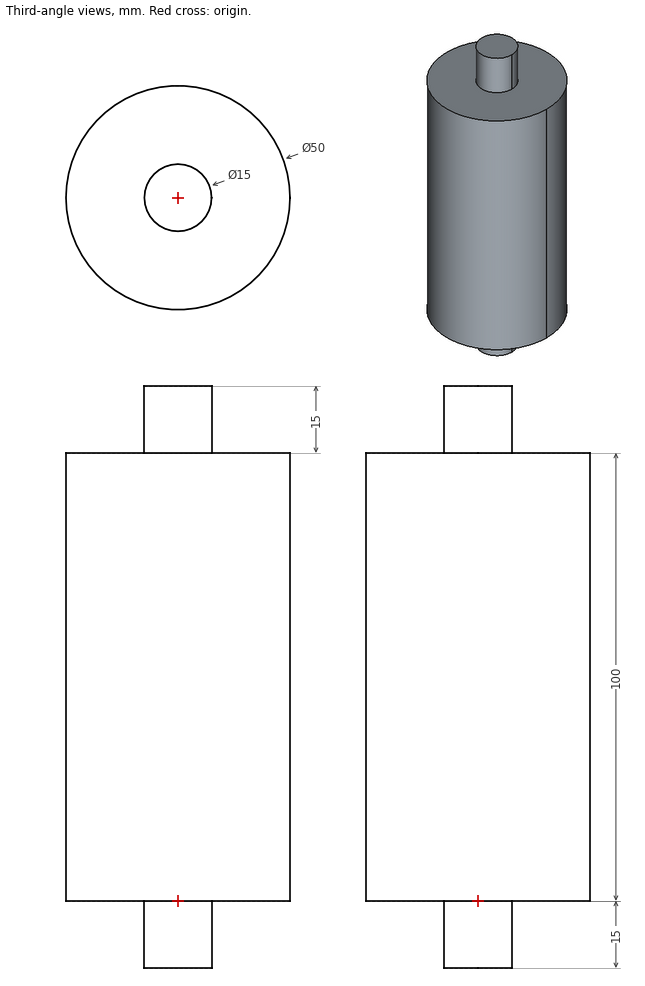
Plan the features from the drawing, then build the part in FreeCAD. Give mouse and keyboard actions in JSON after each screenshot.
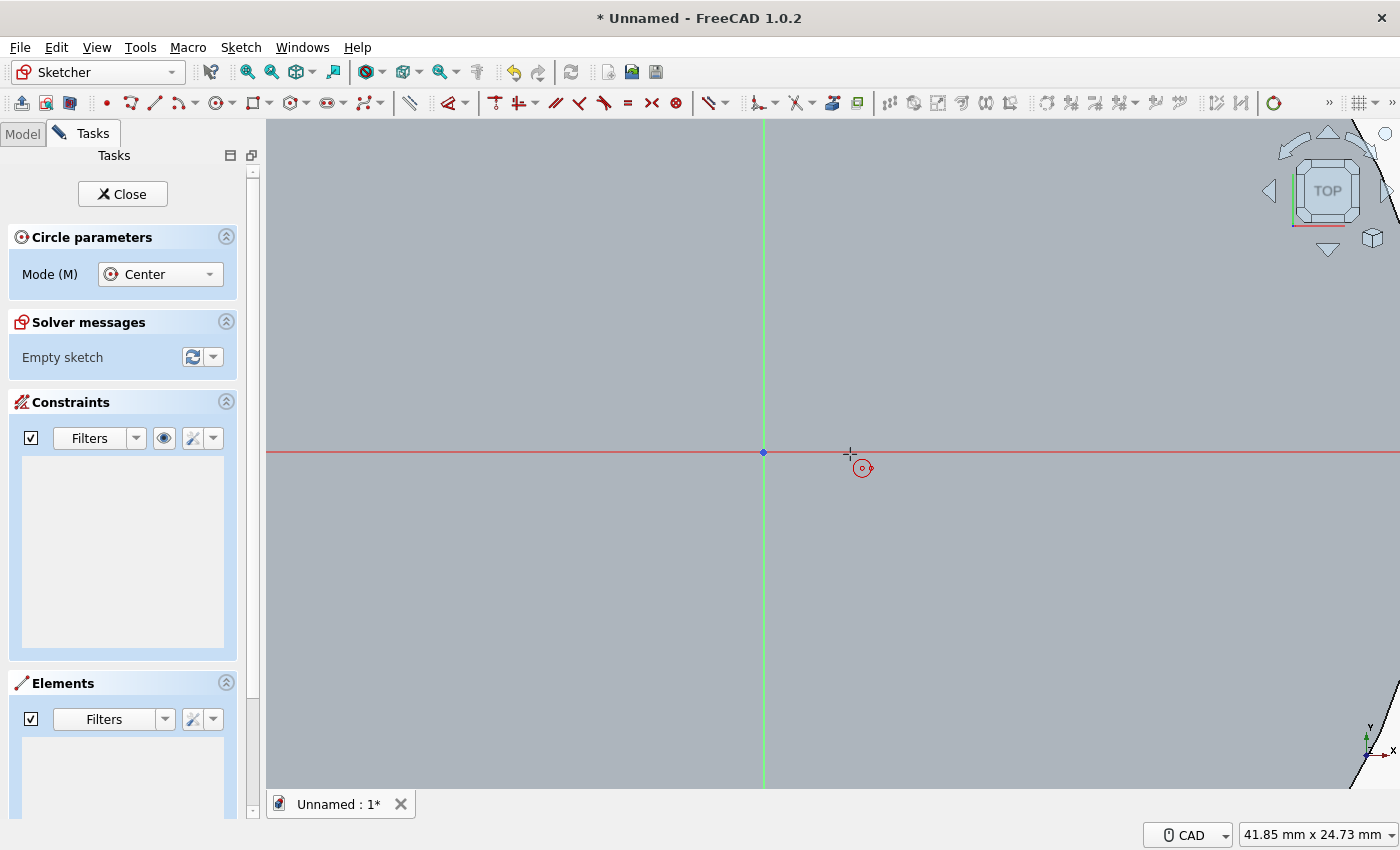
{"action": "left_click", "coordinate": [764, 452]}
{"action": "left_click", "coordinate": [907, 308]}
{"action": "key", "text": "Escape"}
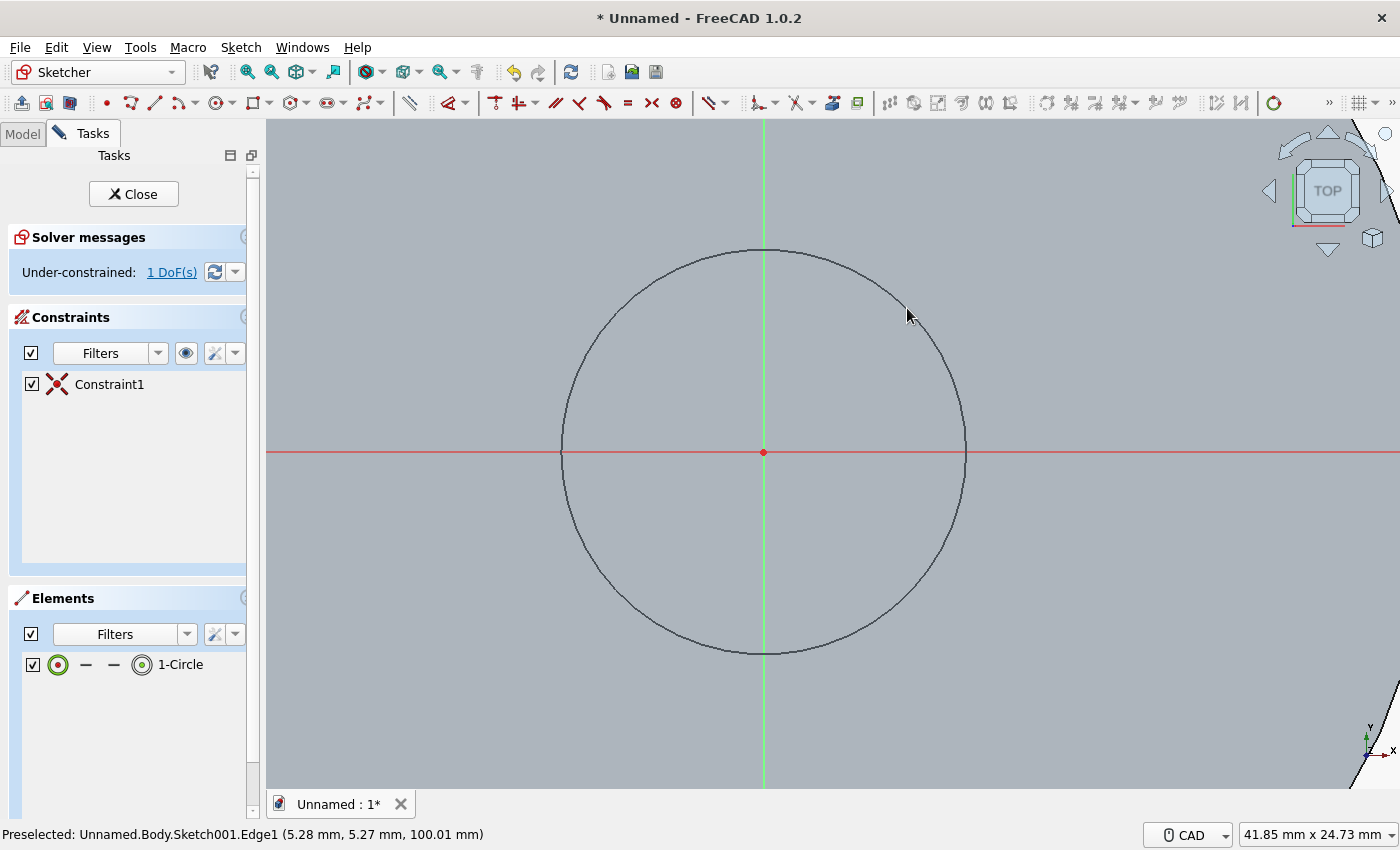
{"action": "left_click", "coordinate": [448, 104]}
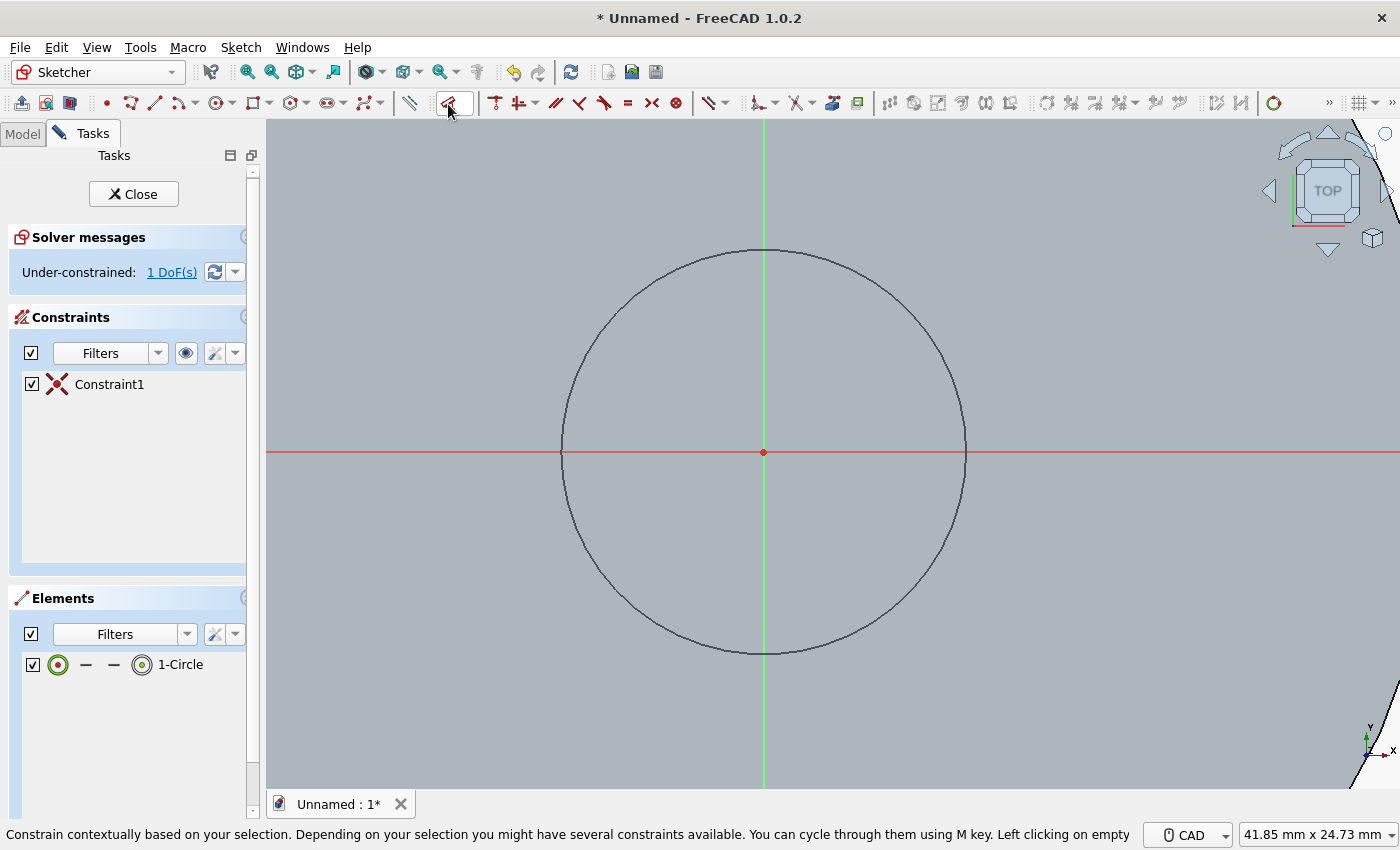
{"action": "left_click", "coordinate": [906, 308]}
{"action": "left_click", "coordinate": [928, 285]}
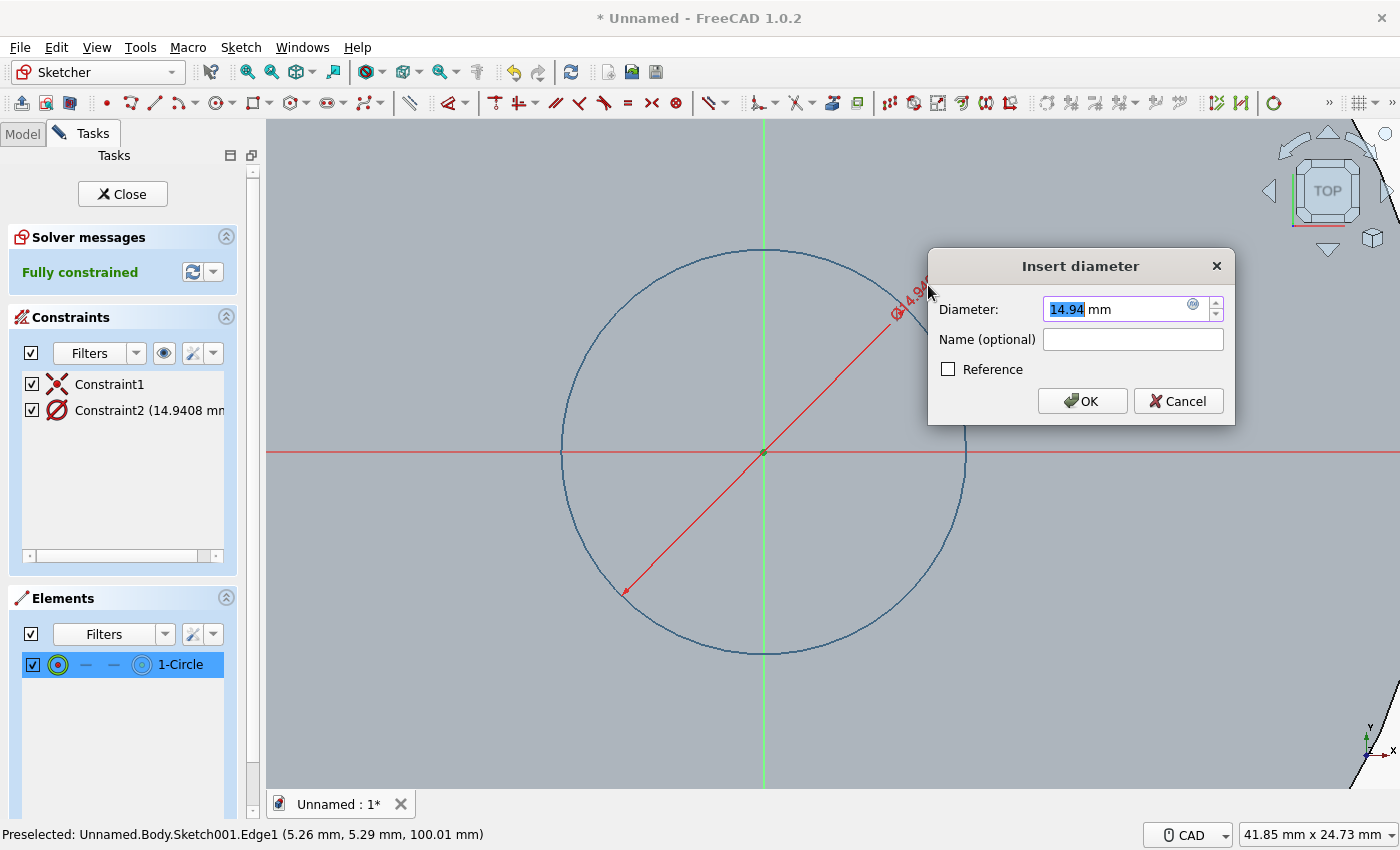
{"action": "type", "text": "15"}
{"action": "key", "text": "Return"}
{"action": "key", "text": "Escape"}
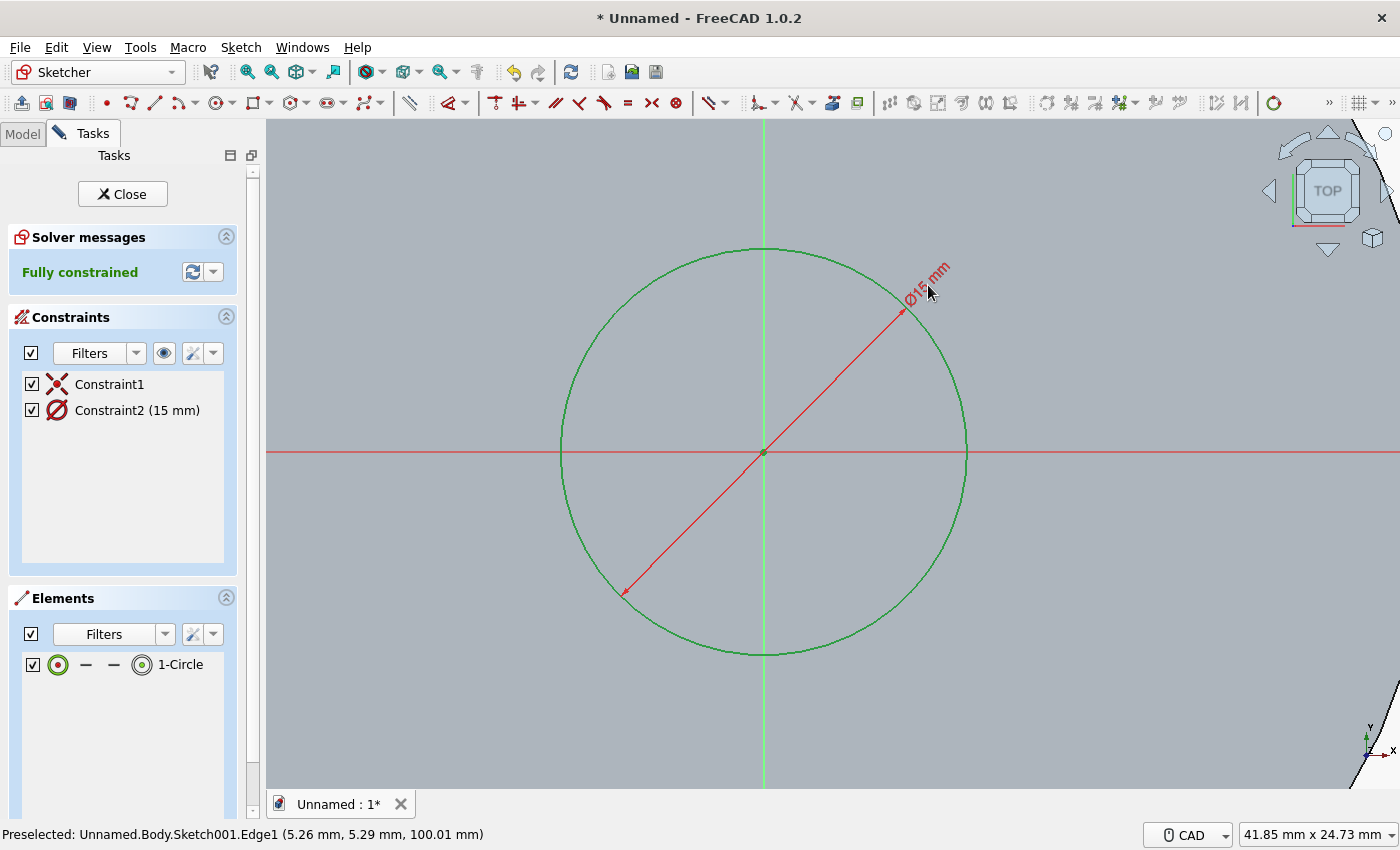
{"action": "left_click", "coordinate": [123, 194]}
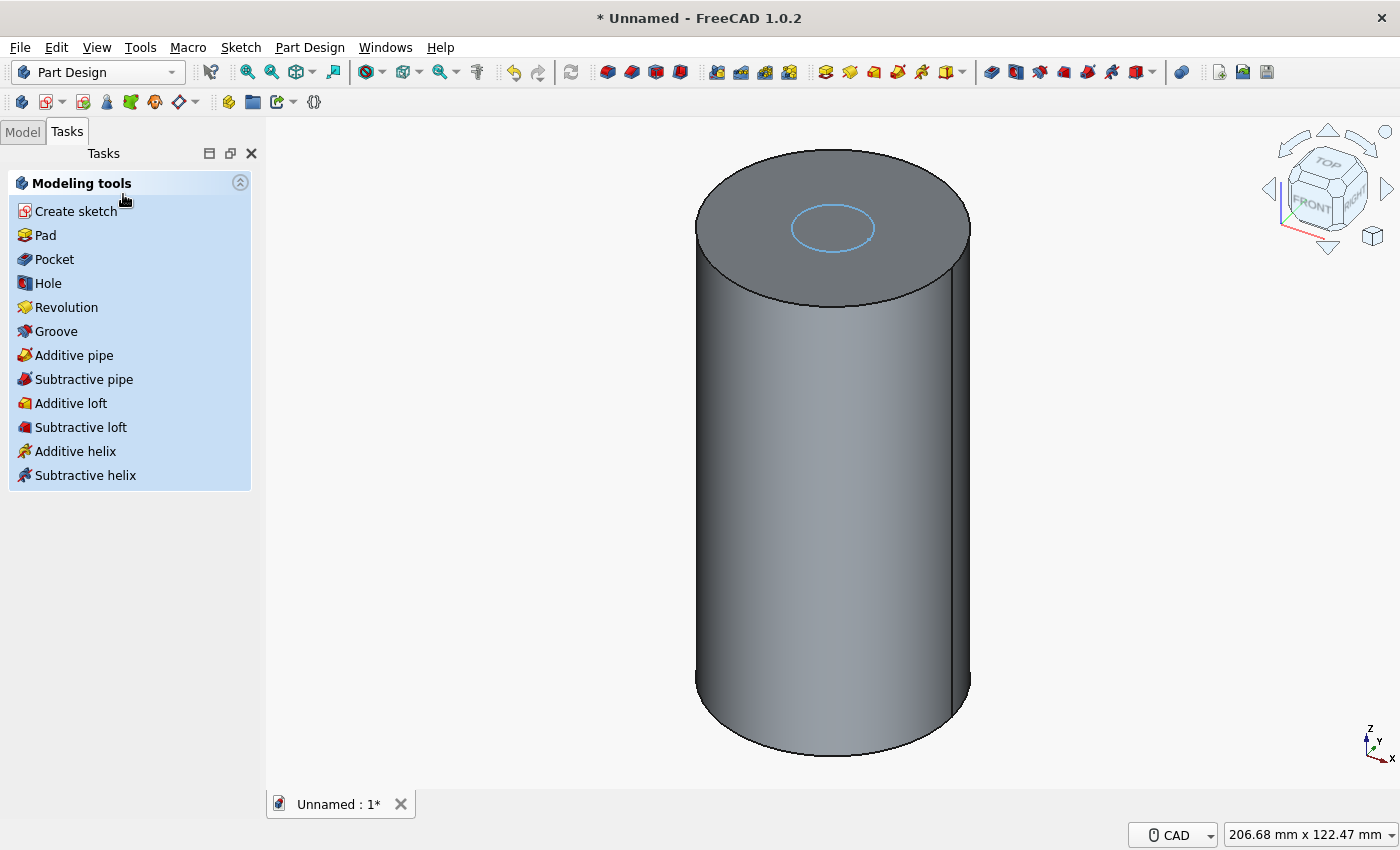
{"action": "left_click", "coordinate": [826, 72]}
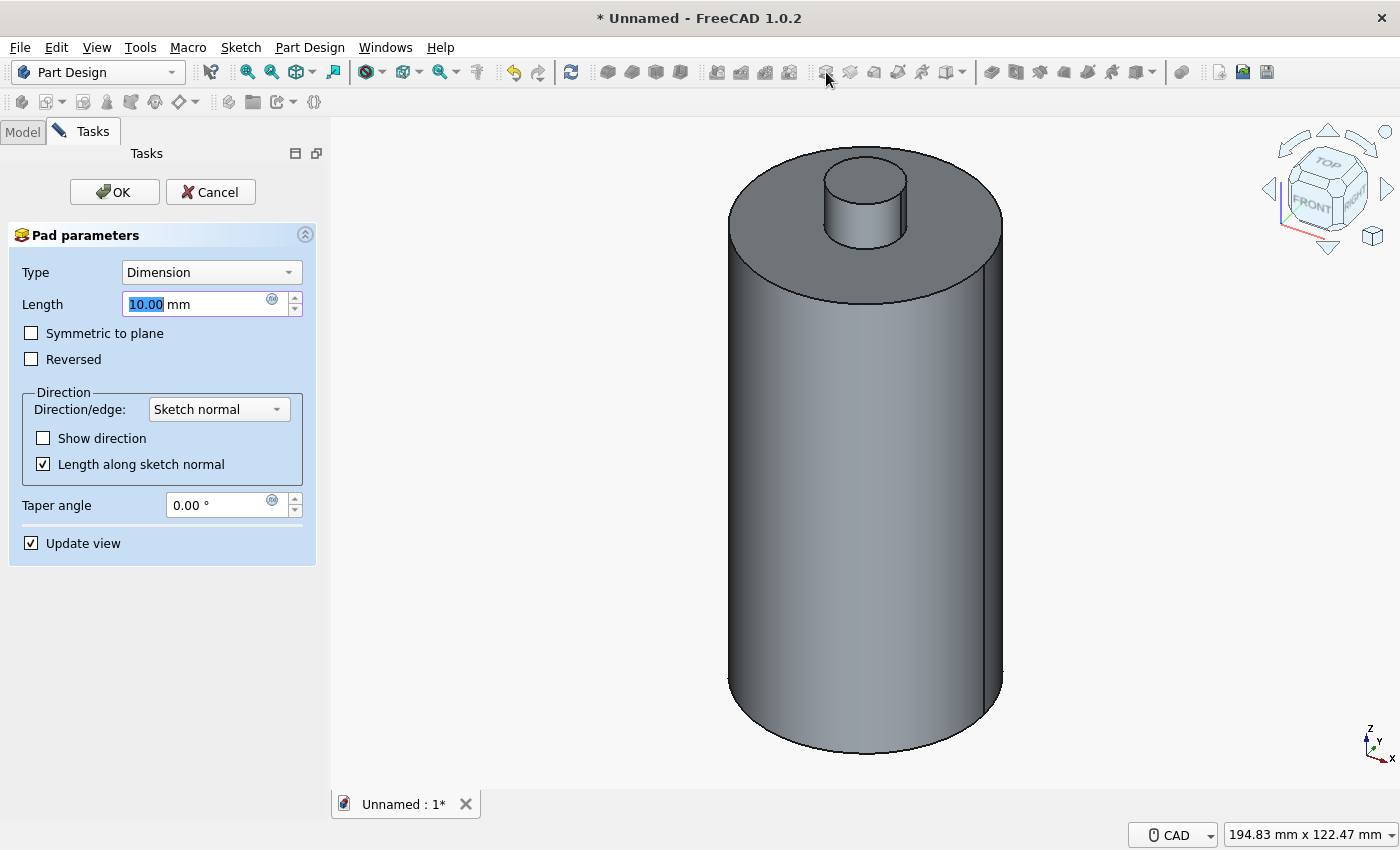
{"action": "type", "text": "15"}
{"action": "key", "text": "Tab"}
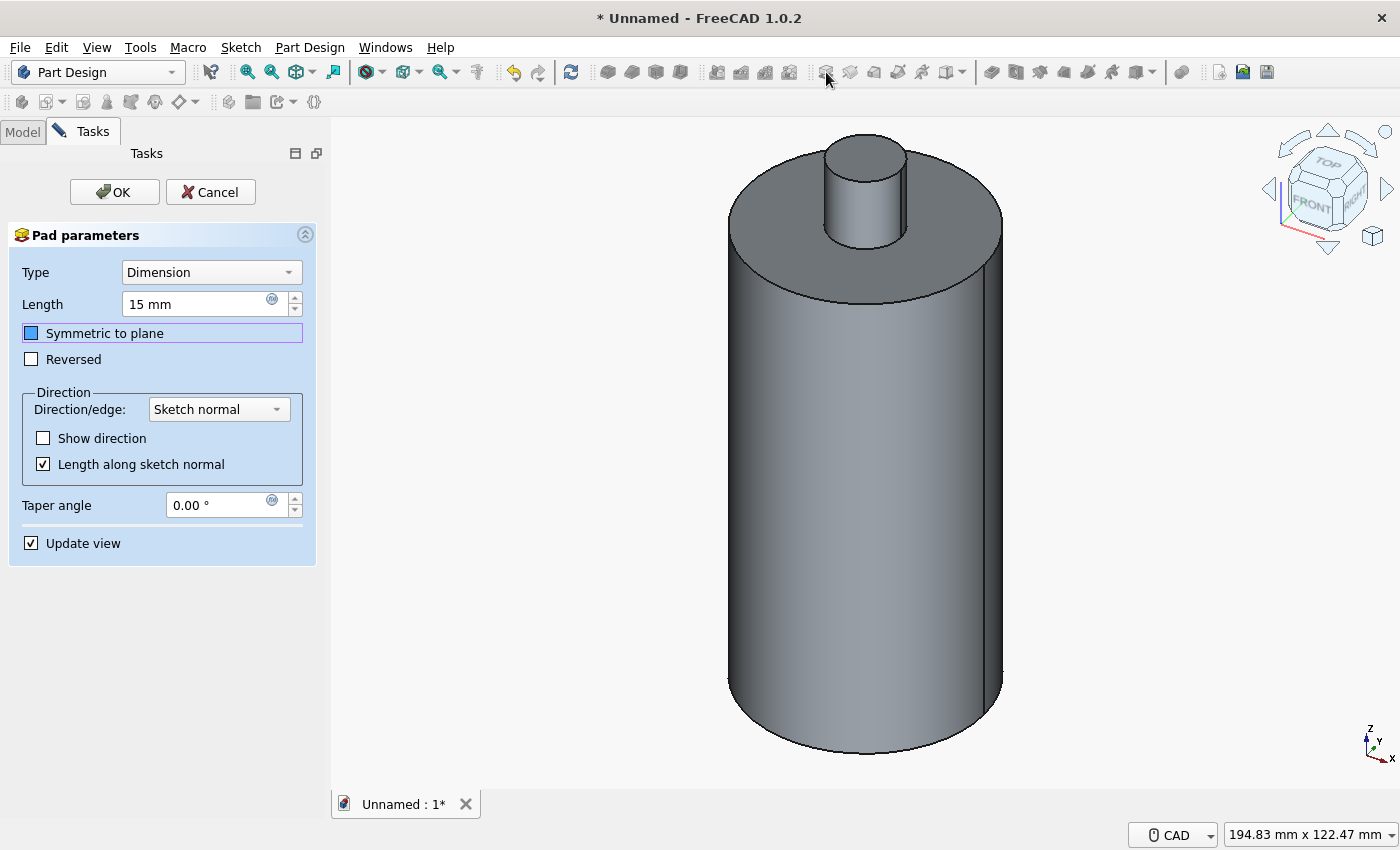
{"action": "left_click", "coordinate": [115, 192]}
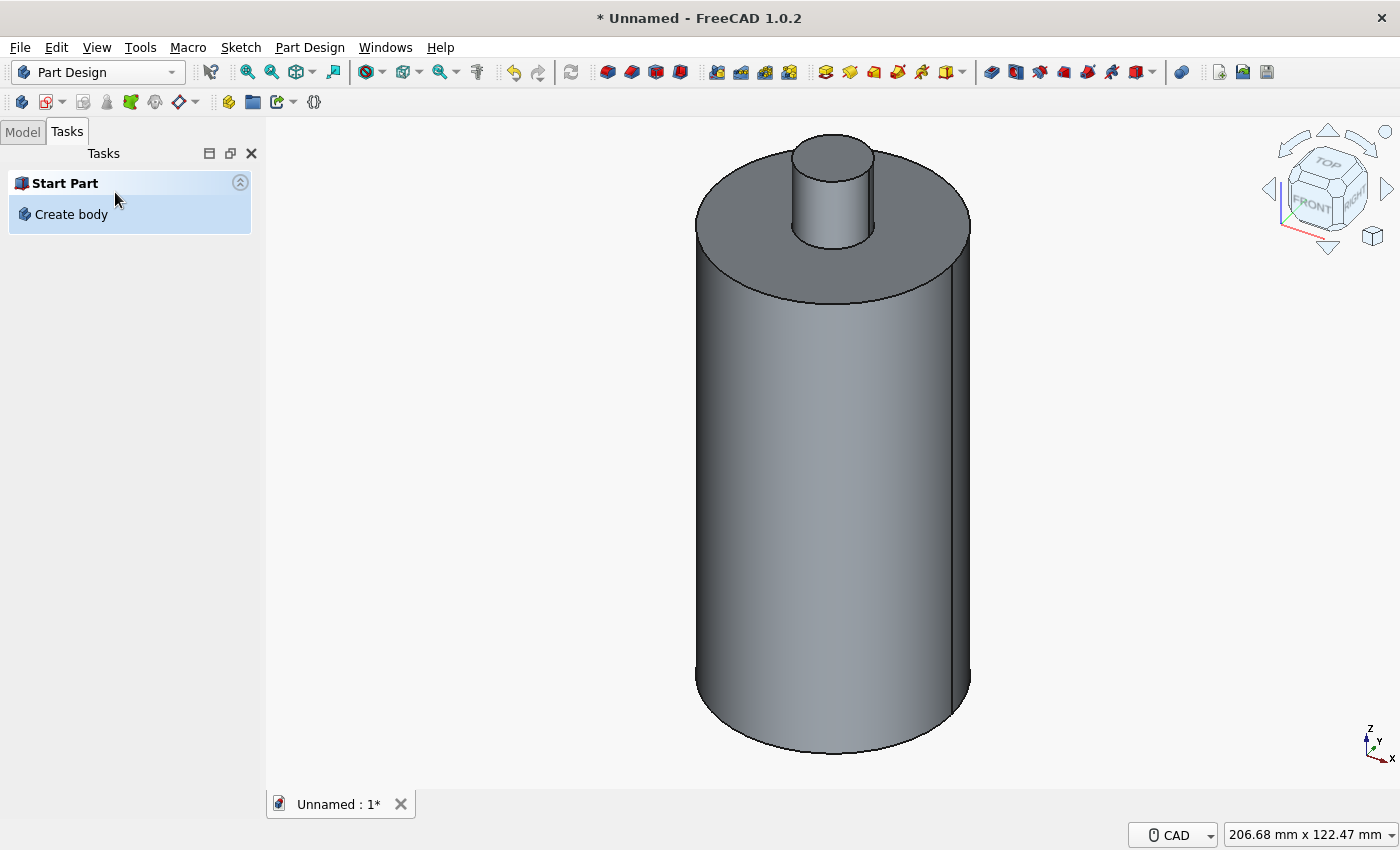
{"action": "key", "text": "v f"}